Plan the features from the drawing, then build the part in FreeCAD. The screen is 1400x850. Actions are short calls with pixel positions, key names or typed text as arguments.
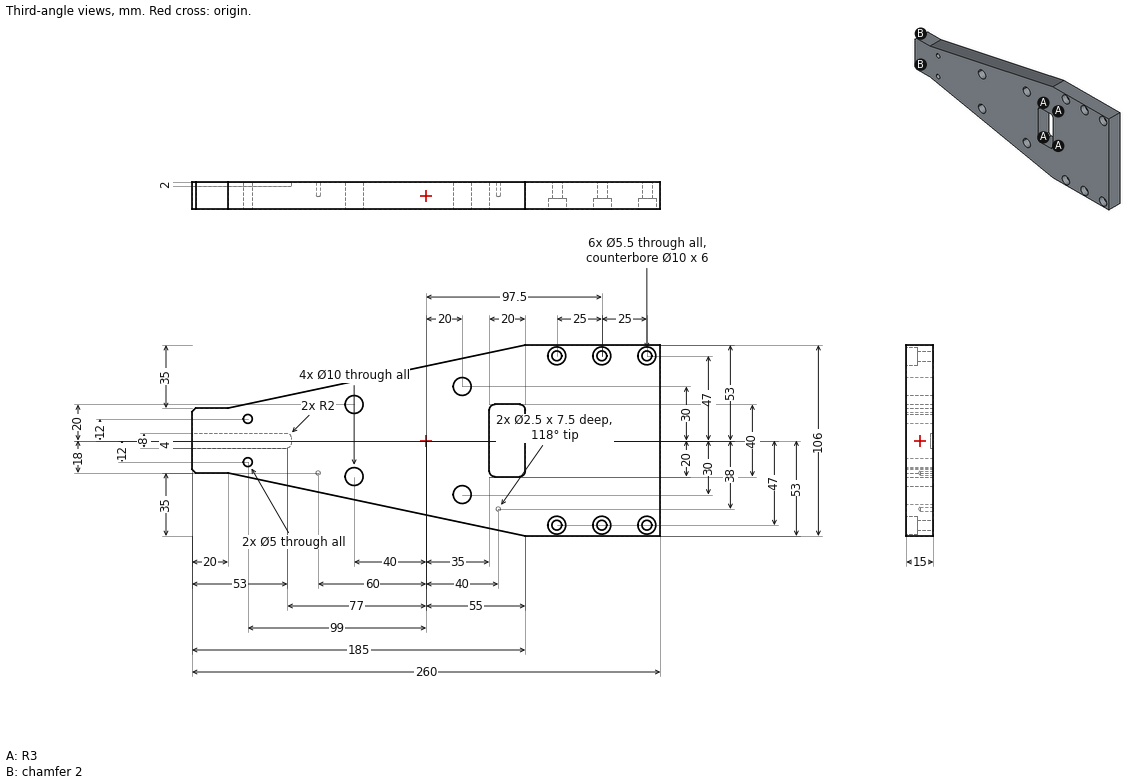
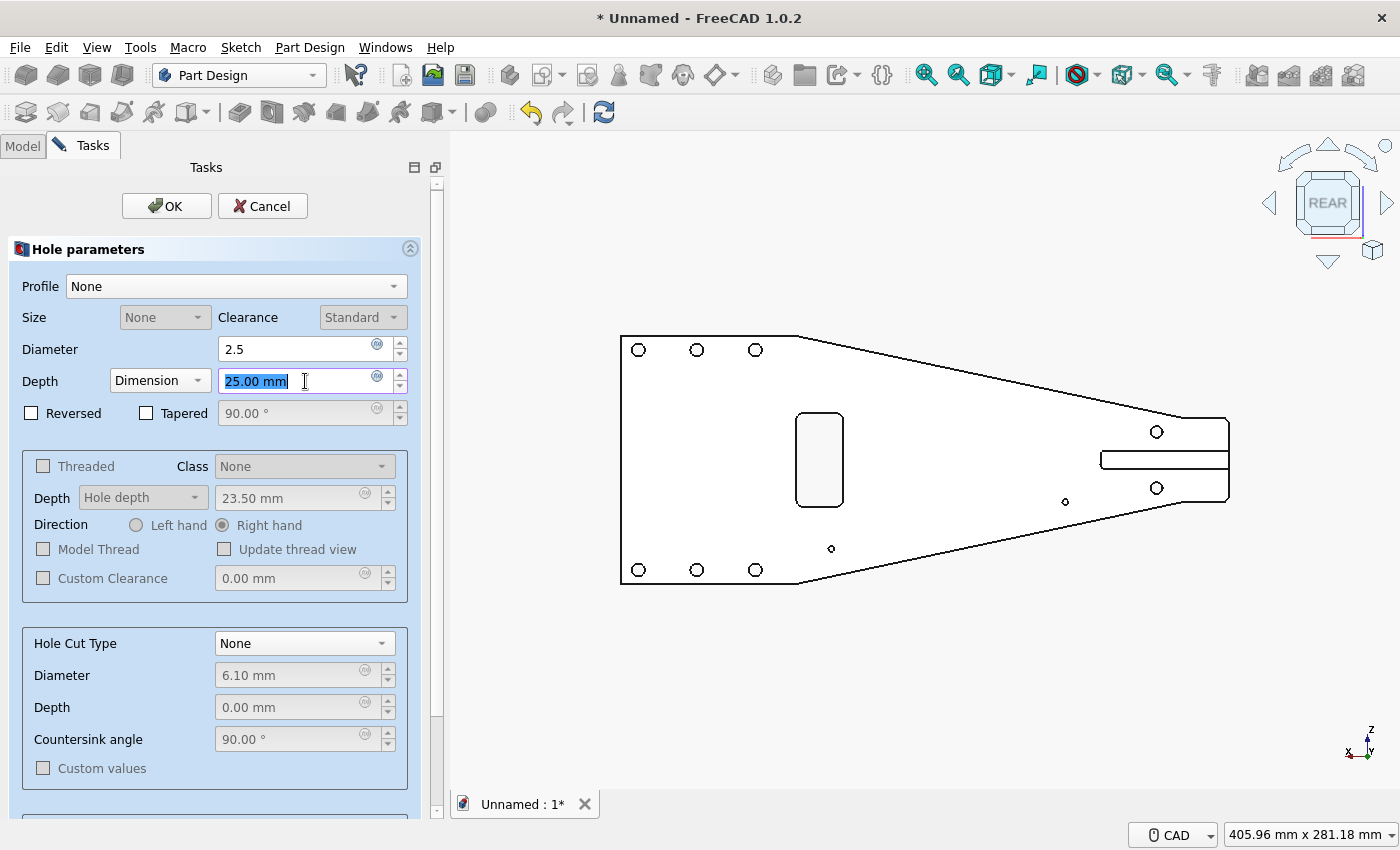
text(7.5)
key(Tab)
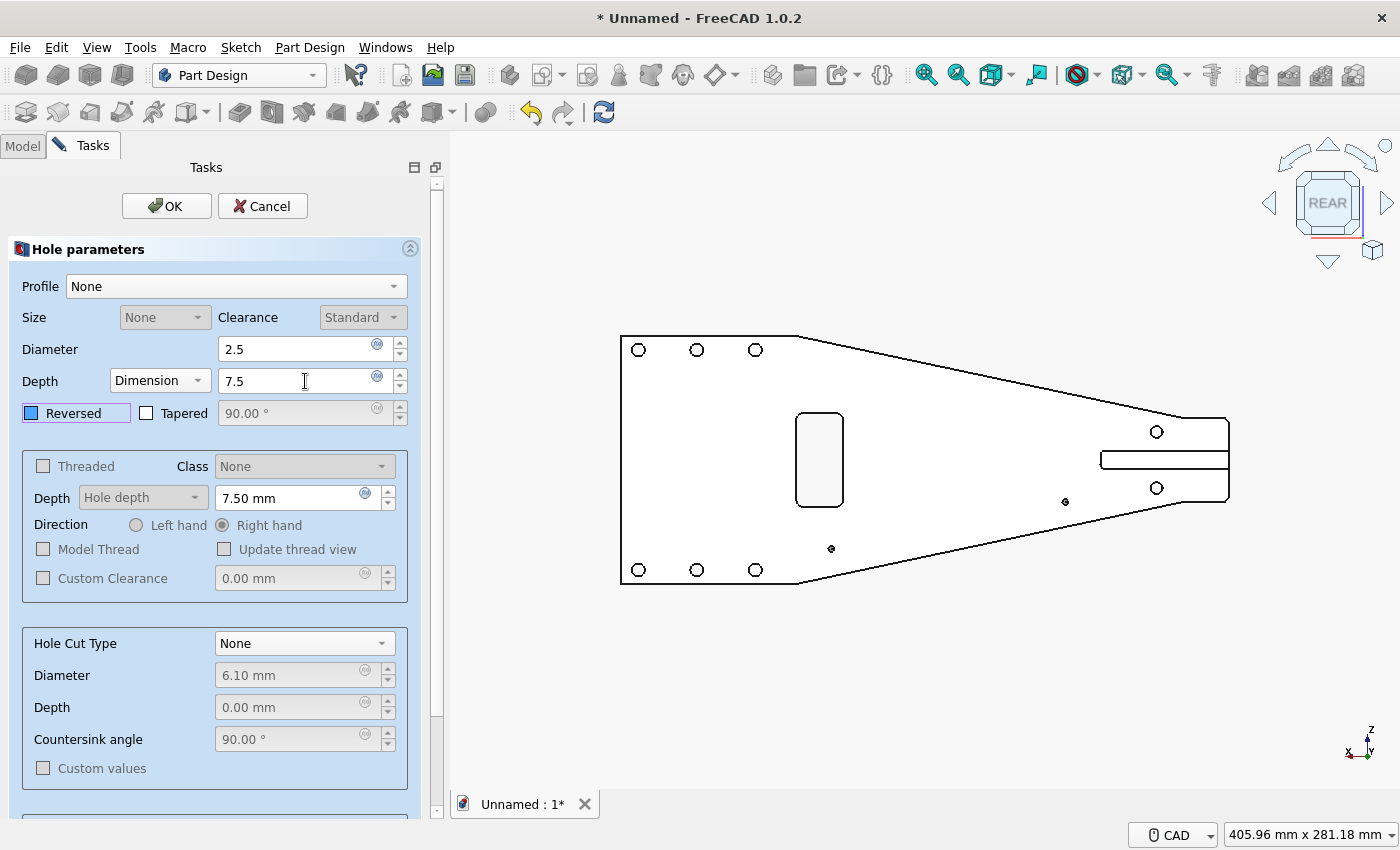
click(167, 206)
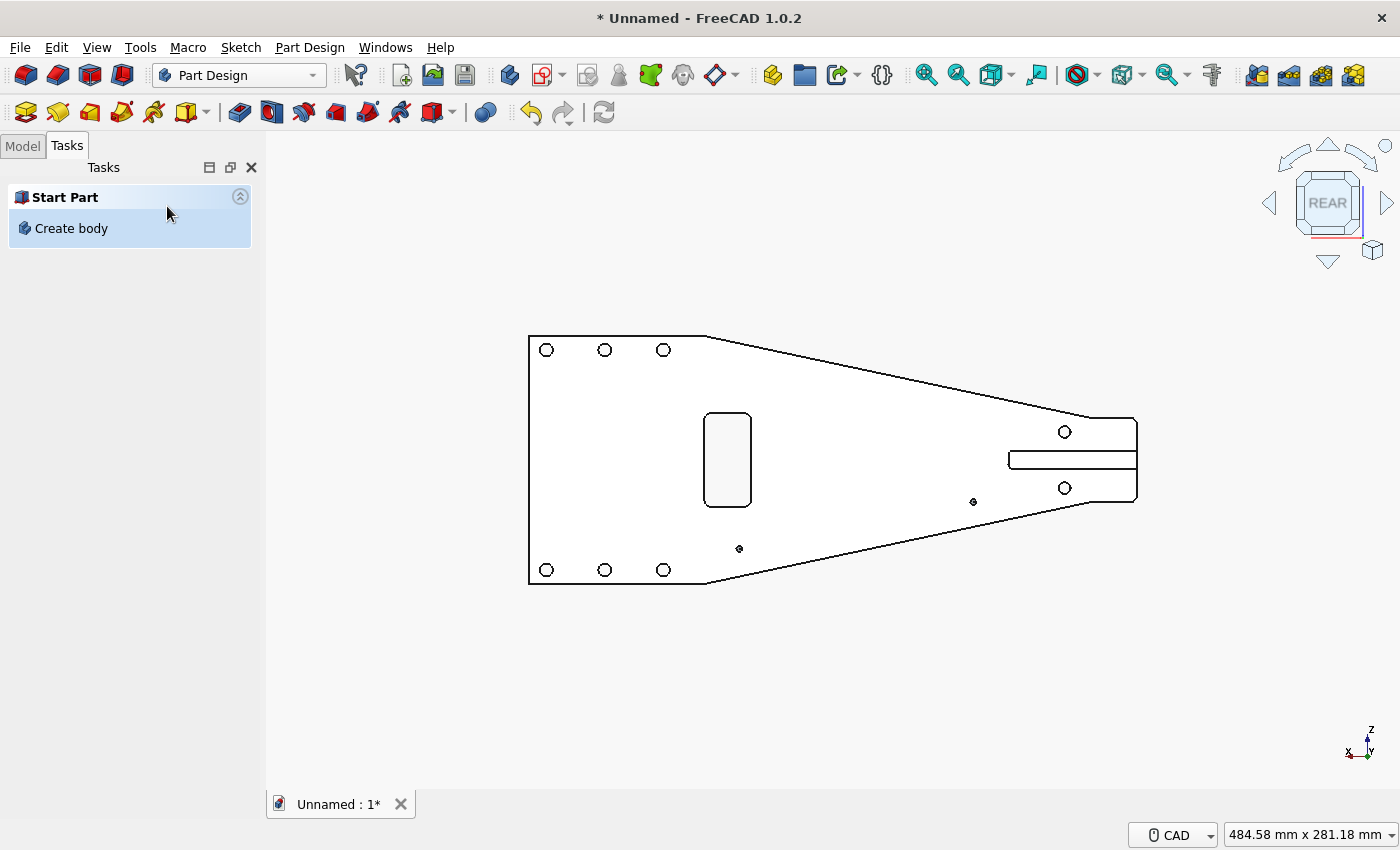
click(833, 459)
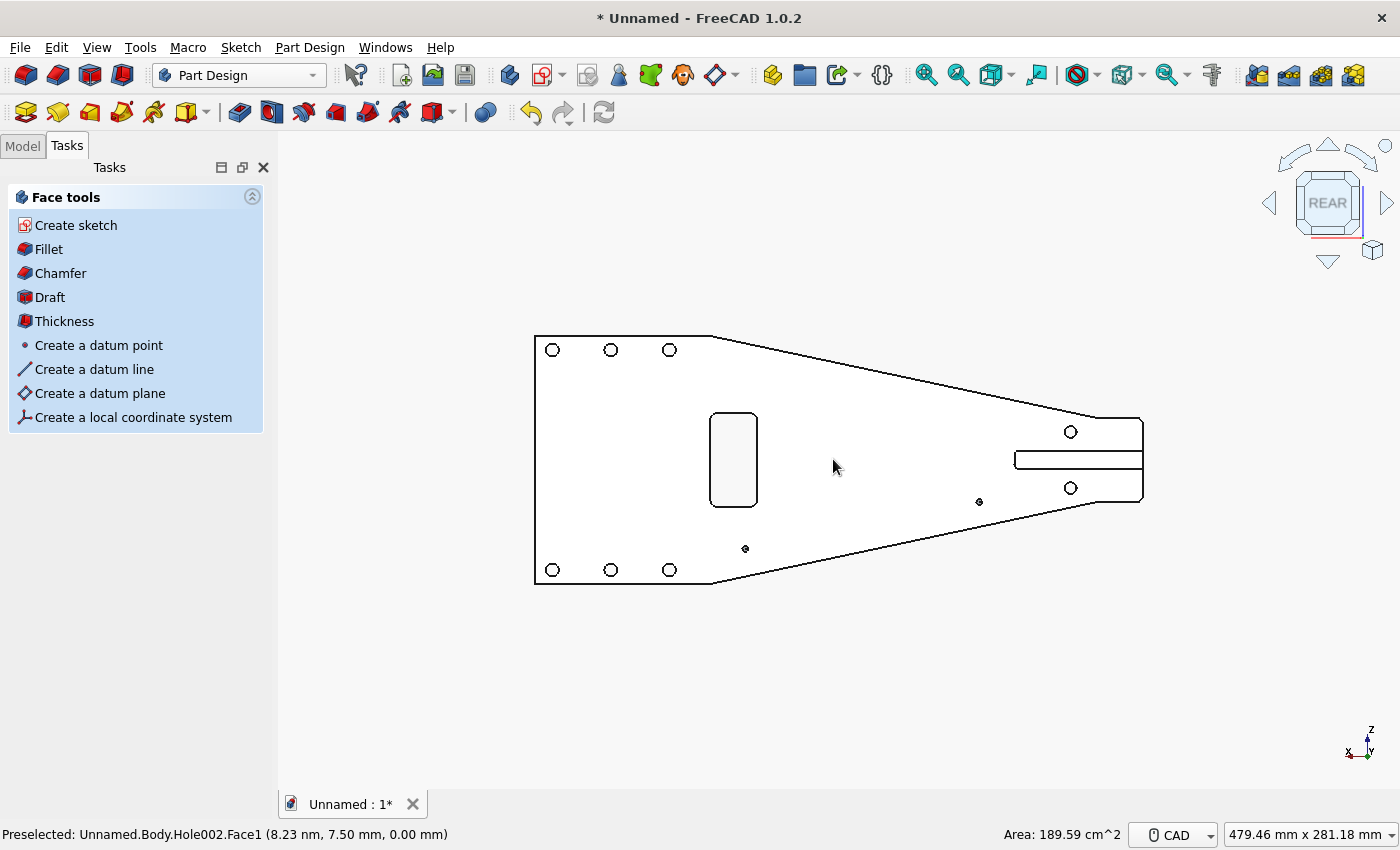
click(542, 76)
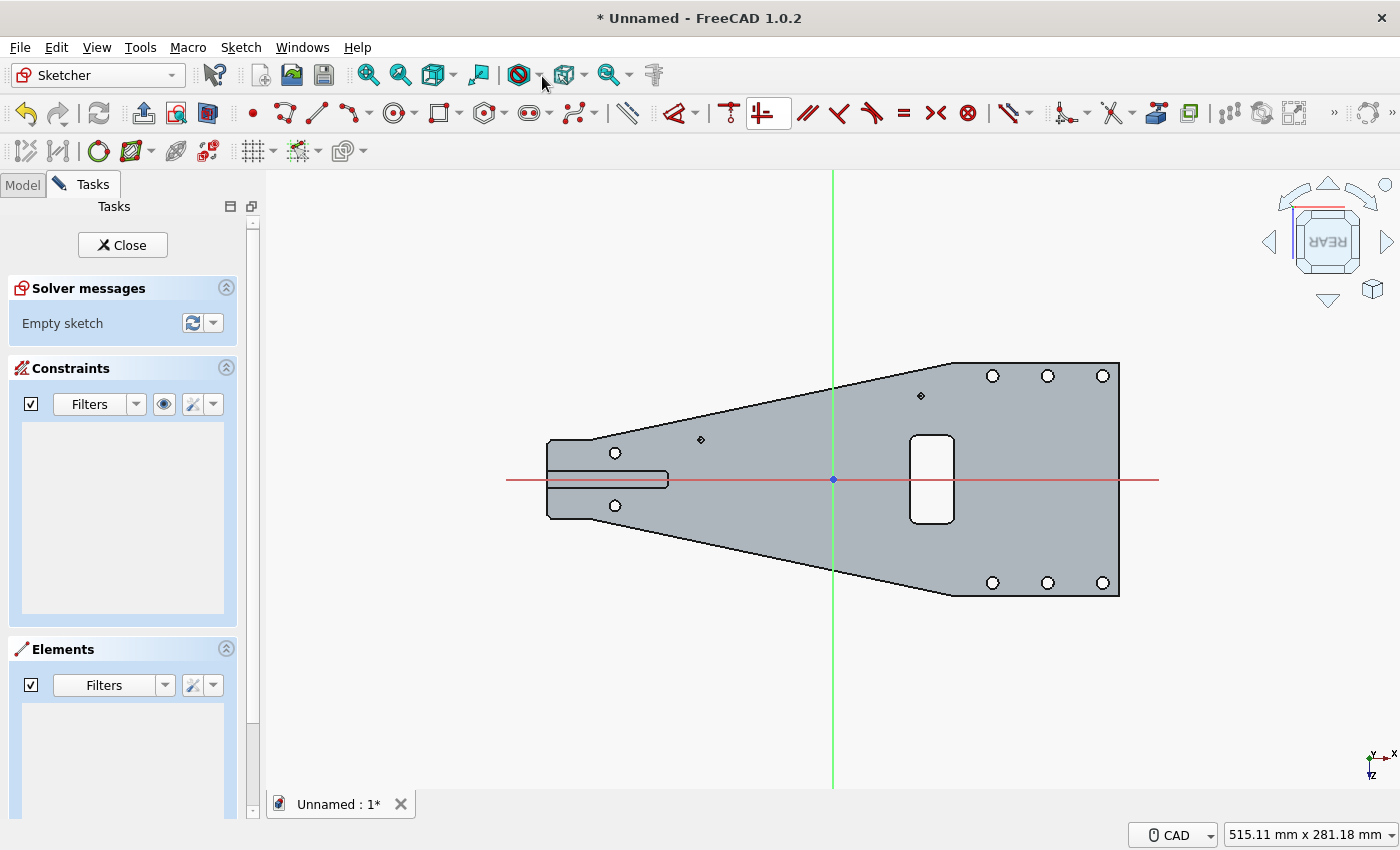
scroll(838, 479, up, 5)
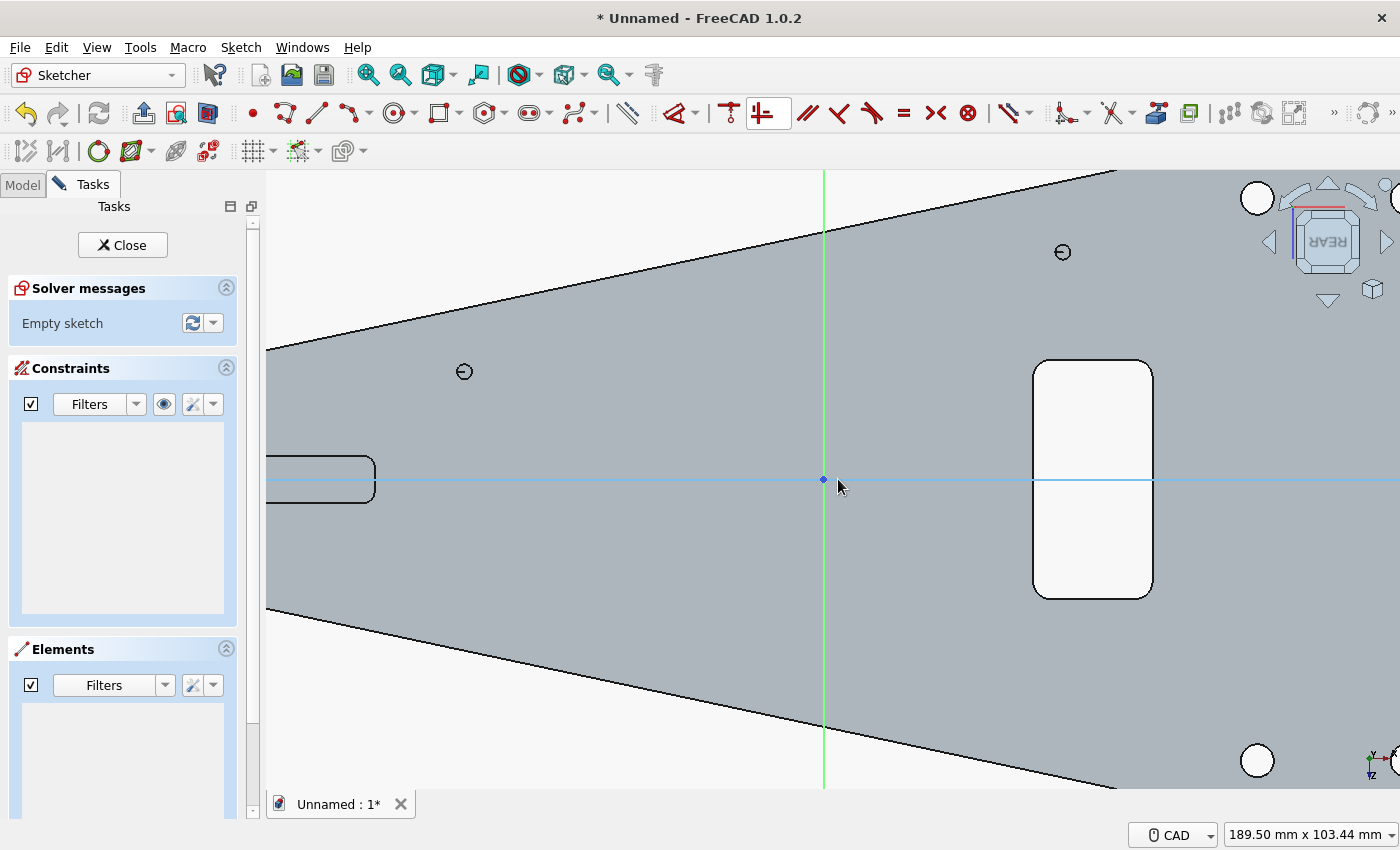
click(394, 114)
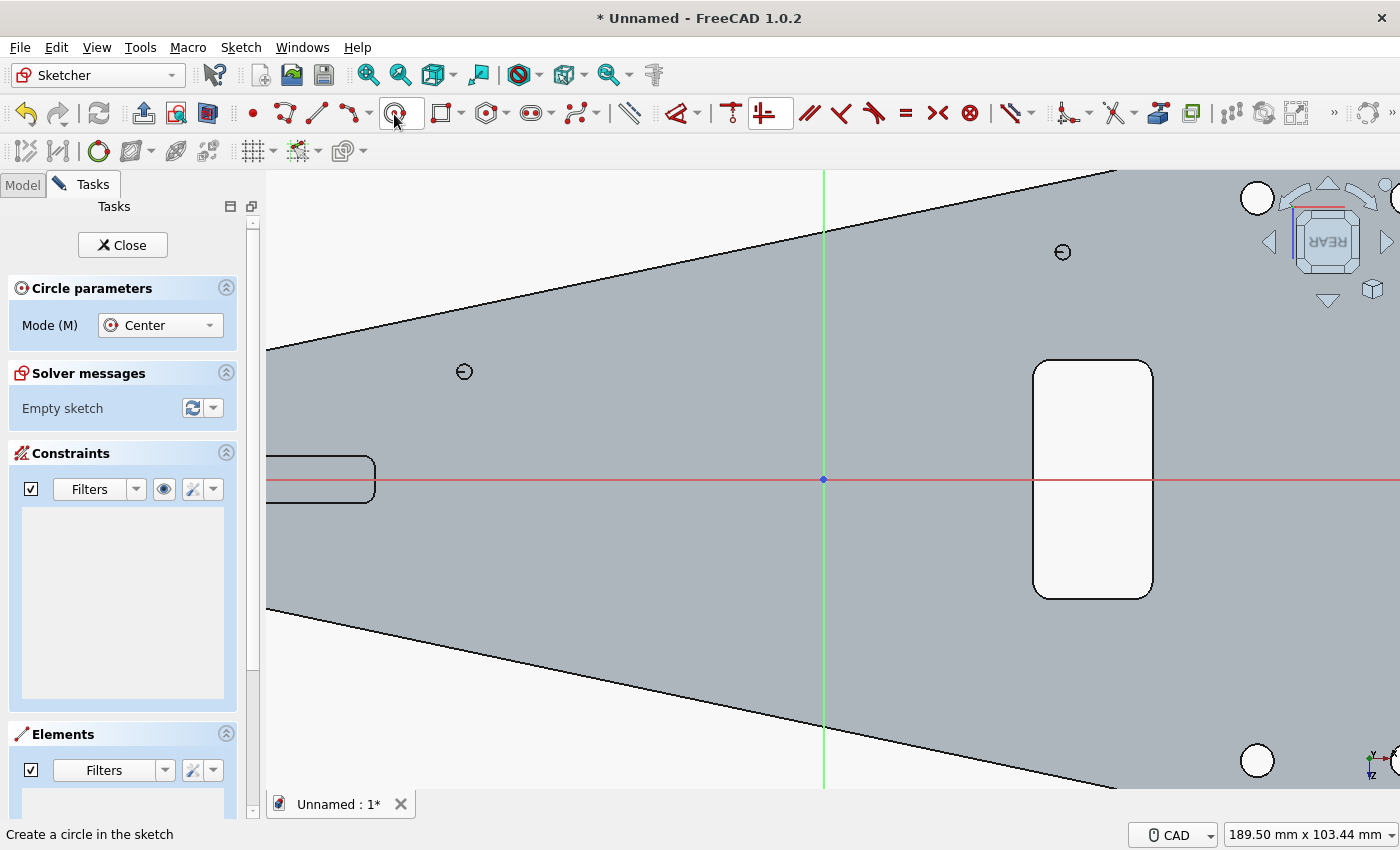
click(584, 360)
click(605, 339)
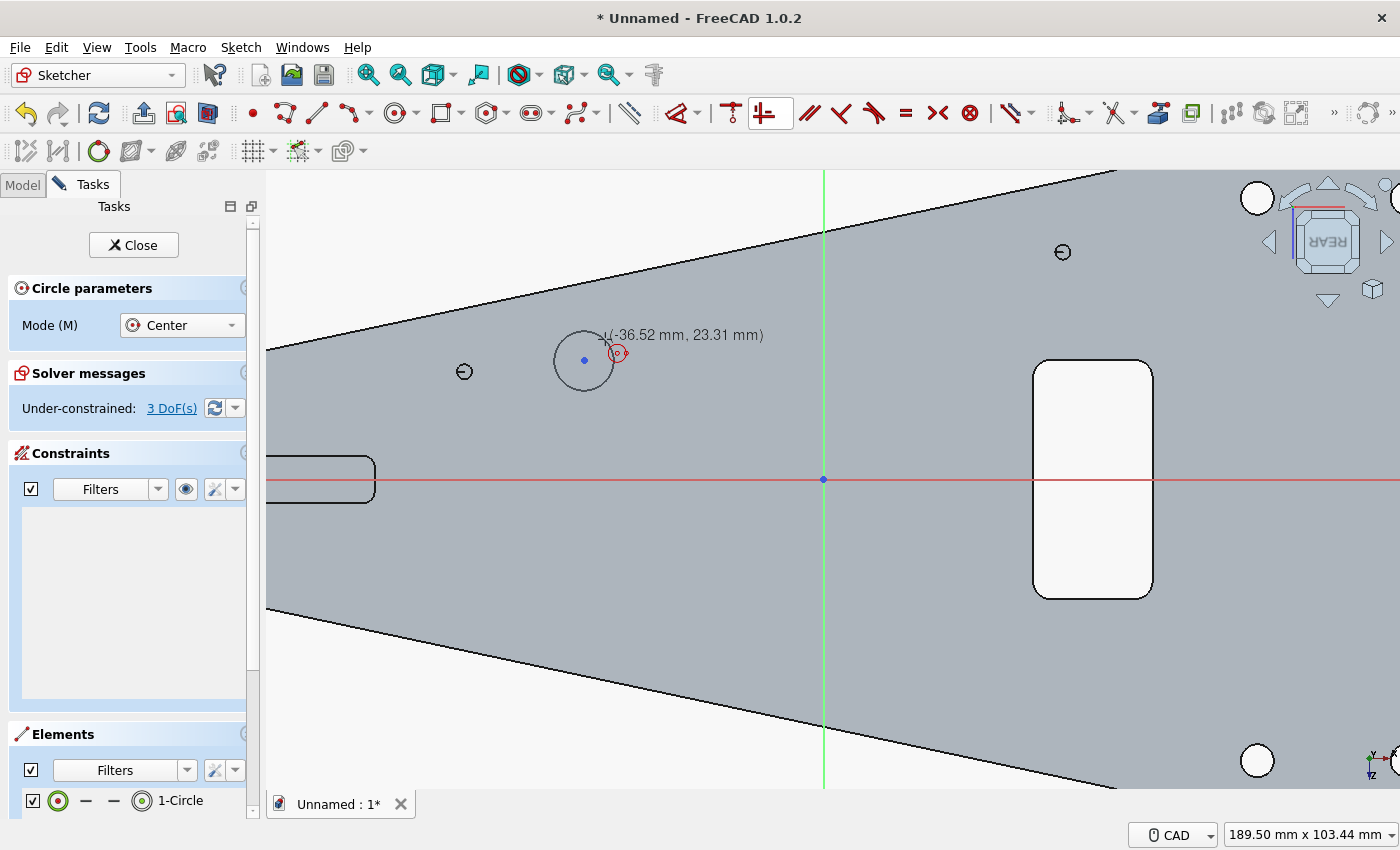
click(584, 599)
click(605, 578)